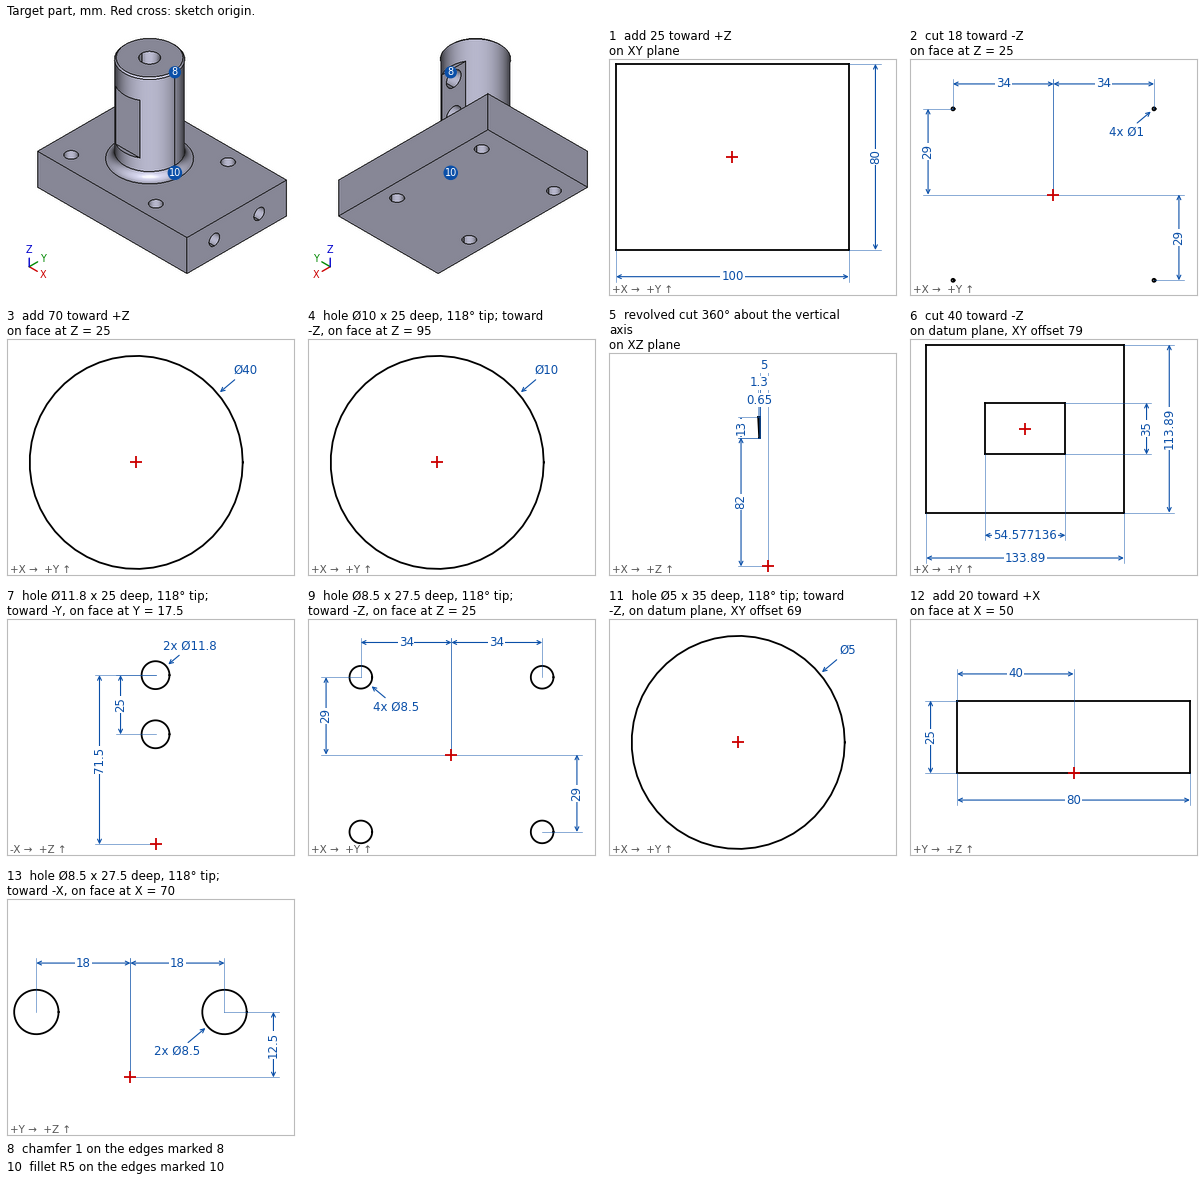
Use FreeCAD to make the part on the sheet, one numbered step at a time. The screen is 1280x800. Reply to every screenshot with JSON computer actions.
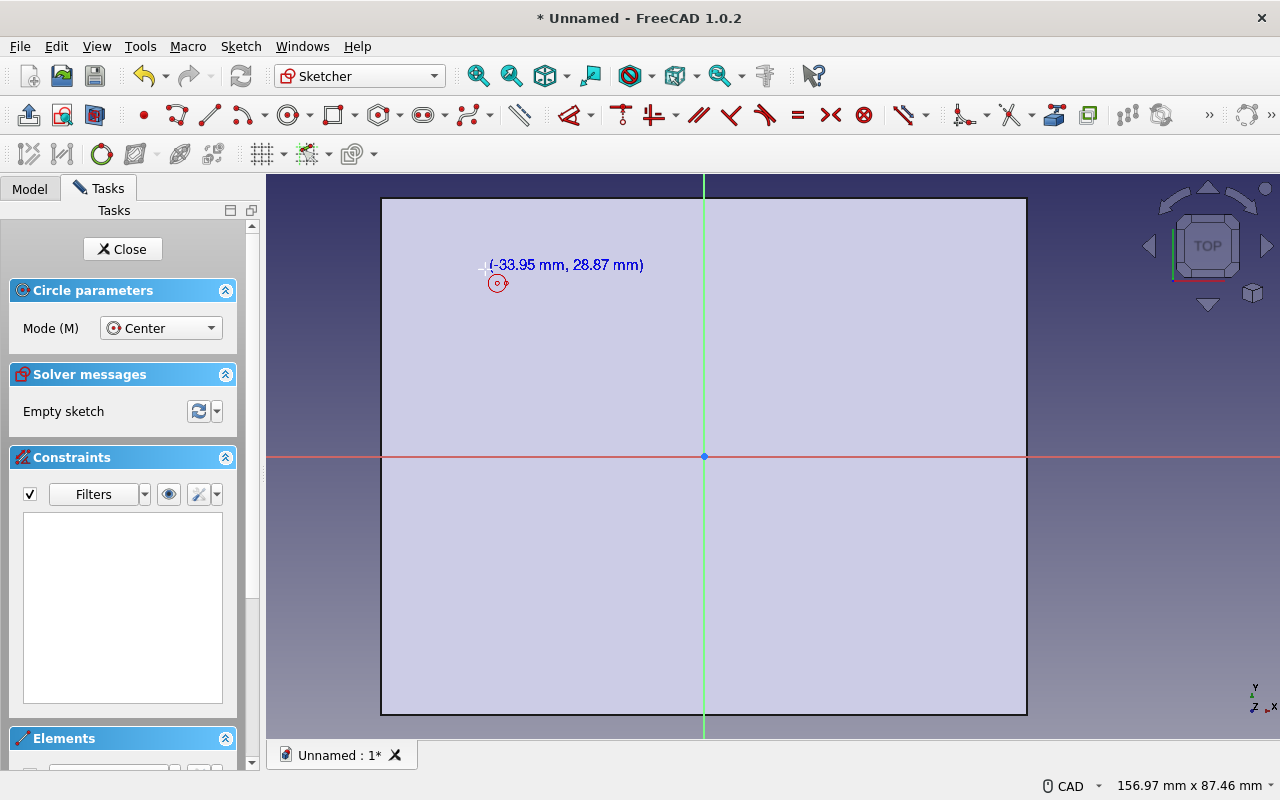
{"action": "left_click", "coordinate": [485, 269]}
{"action": "mouse_move", "coordinate": [487, 267]}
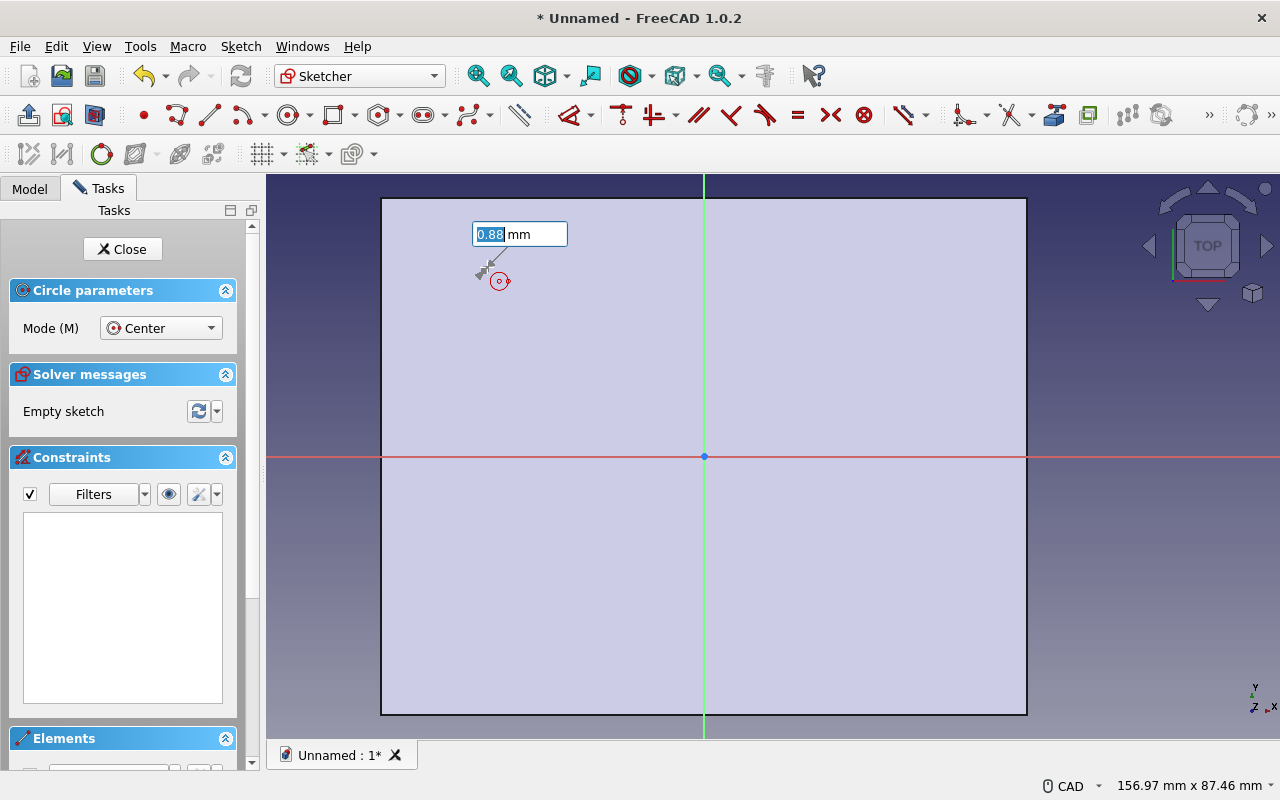
{"action": "type", "text": "1"}
{"action": "key", "text": "Return"}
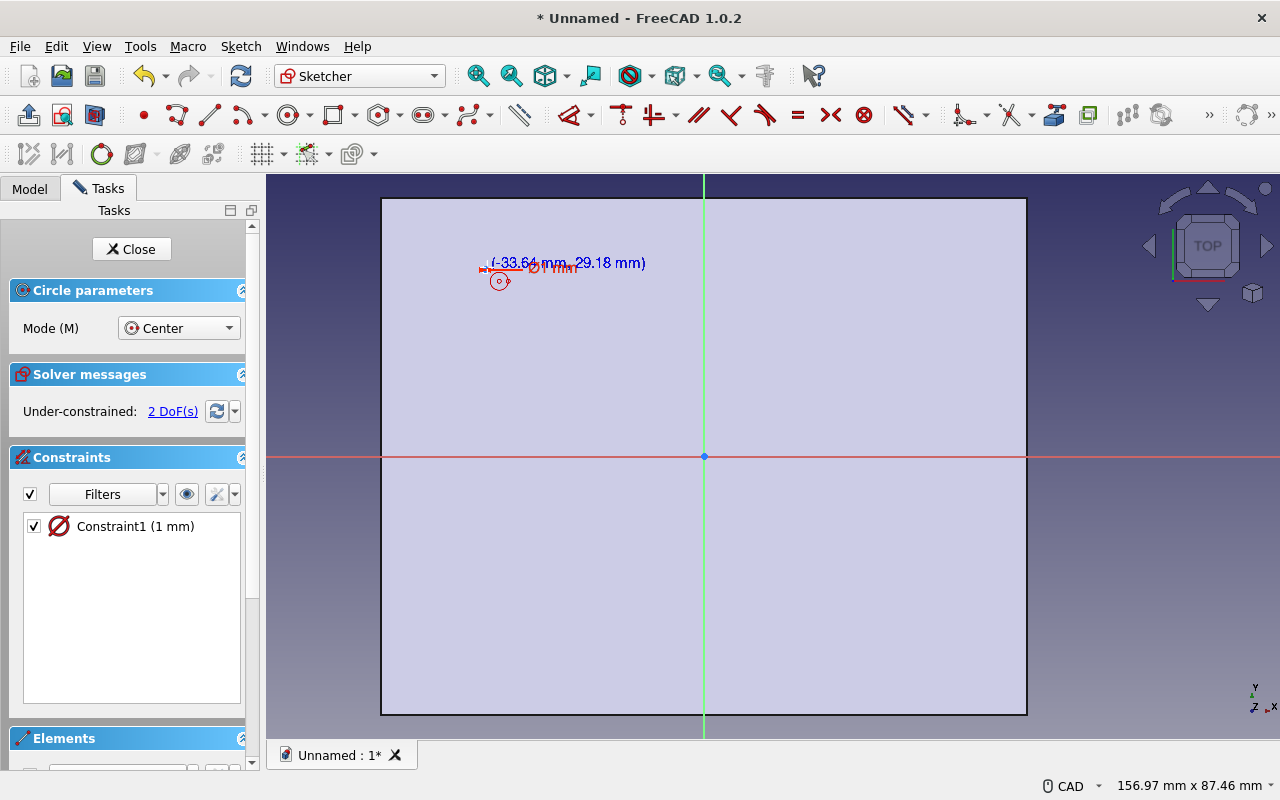
{"action": "scroll", "coordinate": [924, 269], "scroll_direction": "up", "scroll_amount": 10}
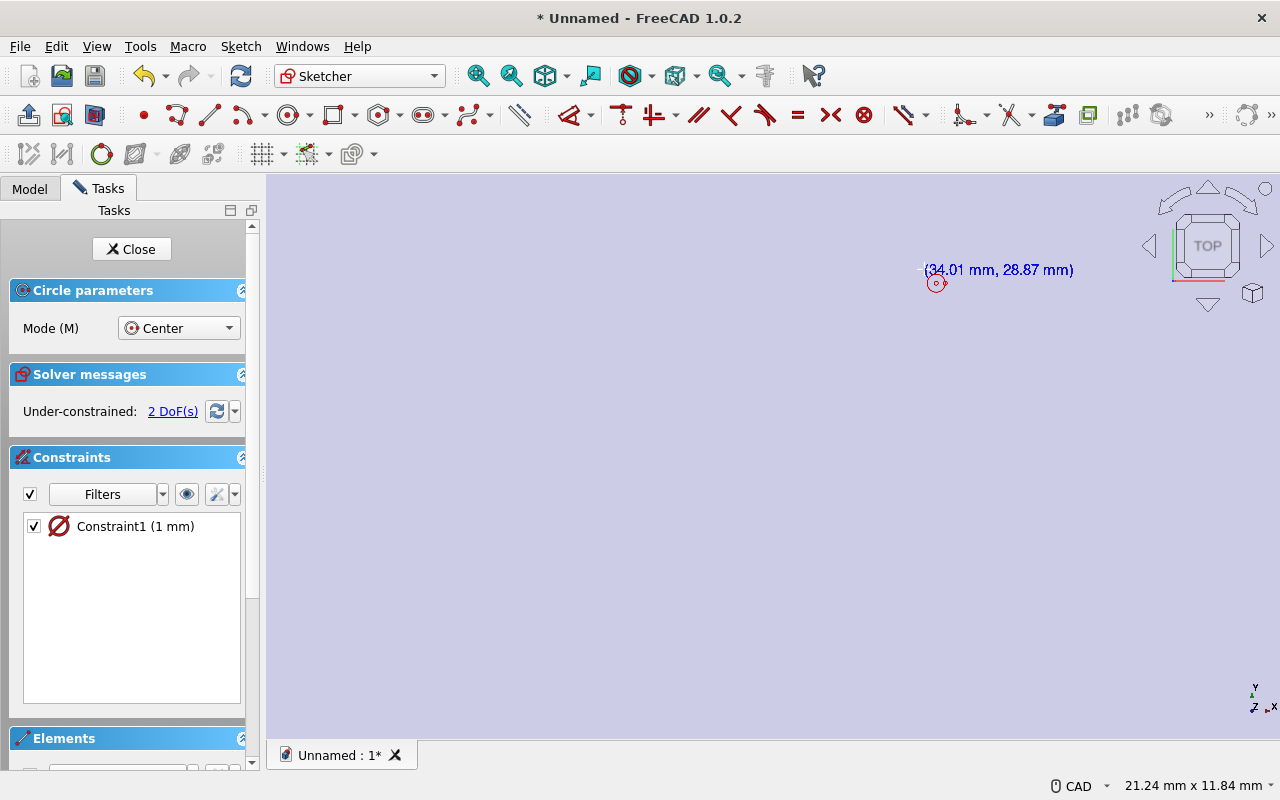
{"action": "scroll", "coordinate": [925, 269], "scroll_direction": "down", "scroll_amount": 10}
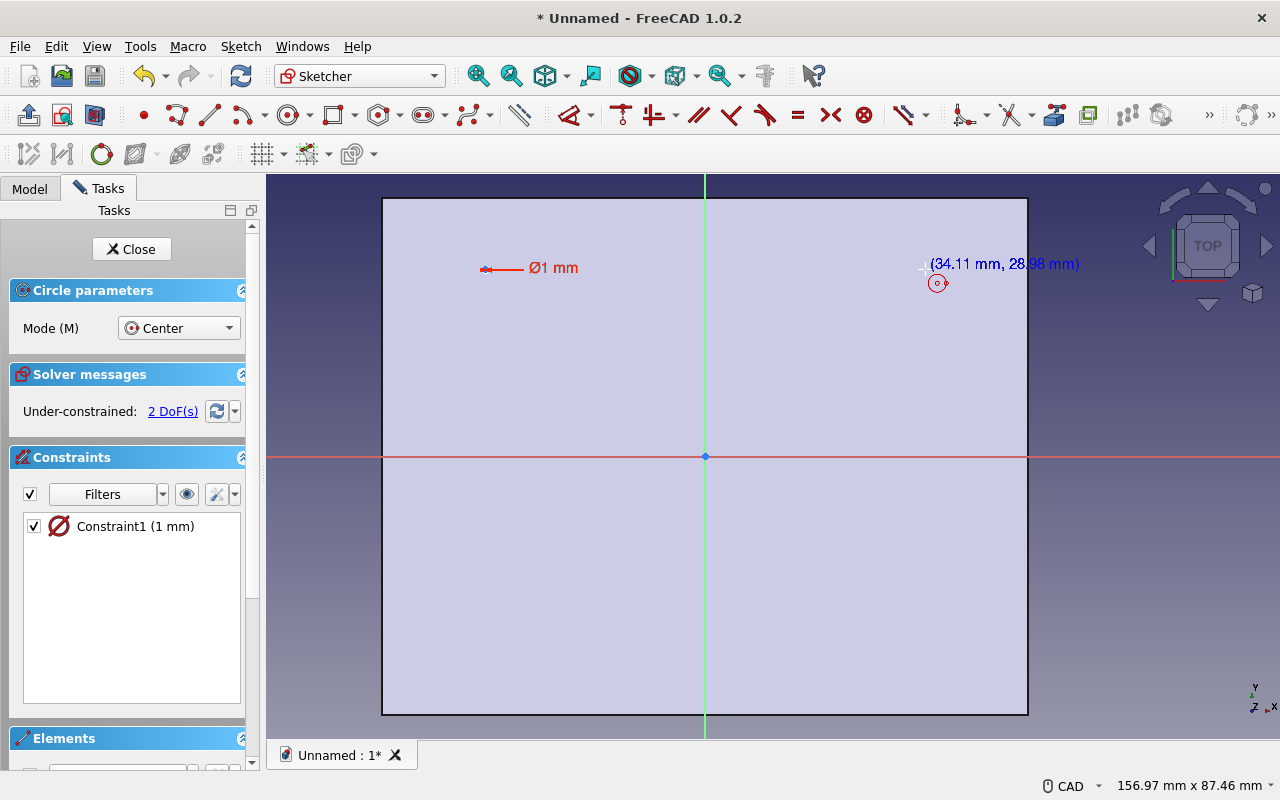
{"action": "left_click", "coordinate": [925, 269]}
{"action": "mouse_move", "coordinate": [927, 267]}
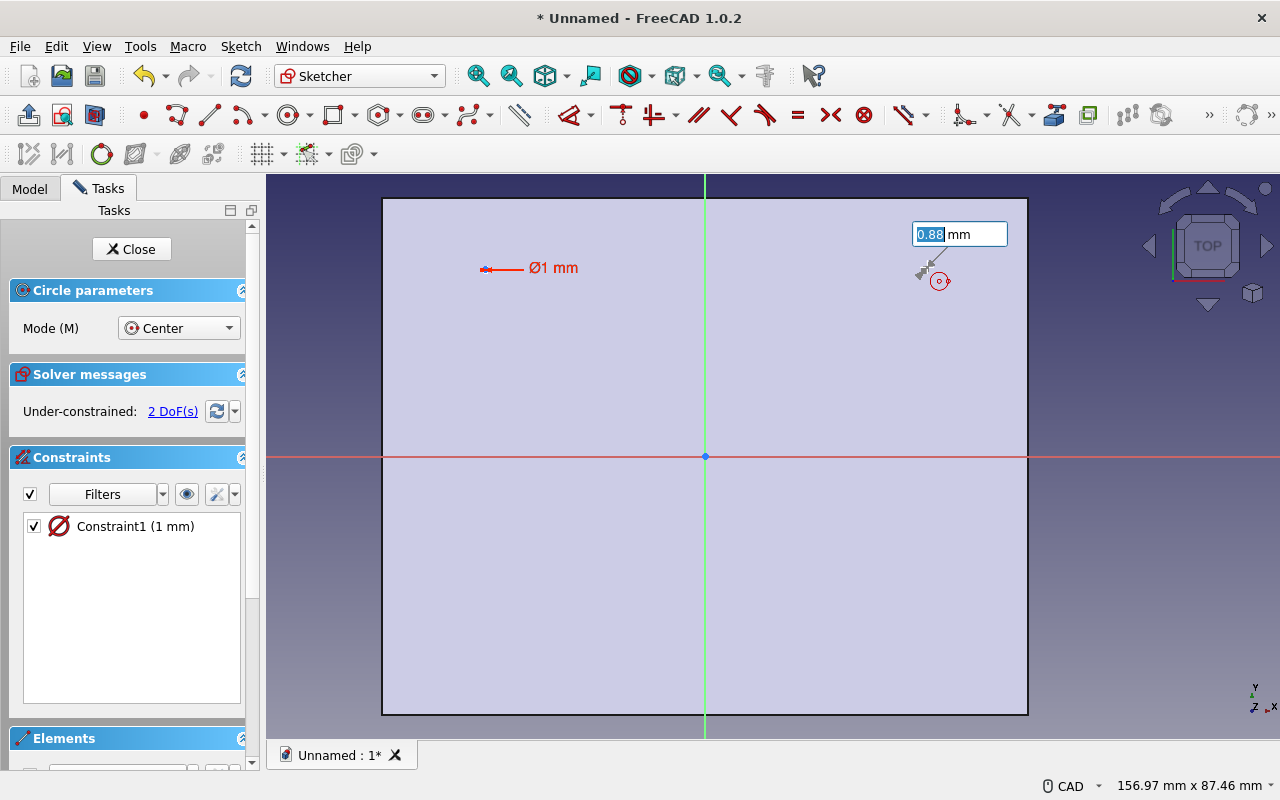
{"action": "type", "text": "1"}
{"action": "key", "text": "Return"}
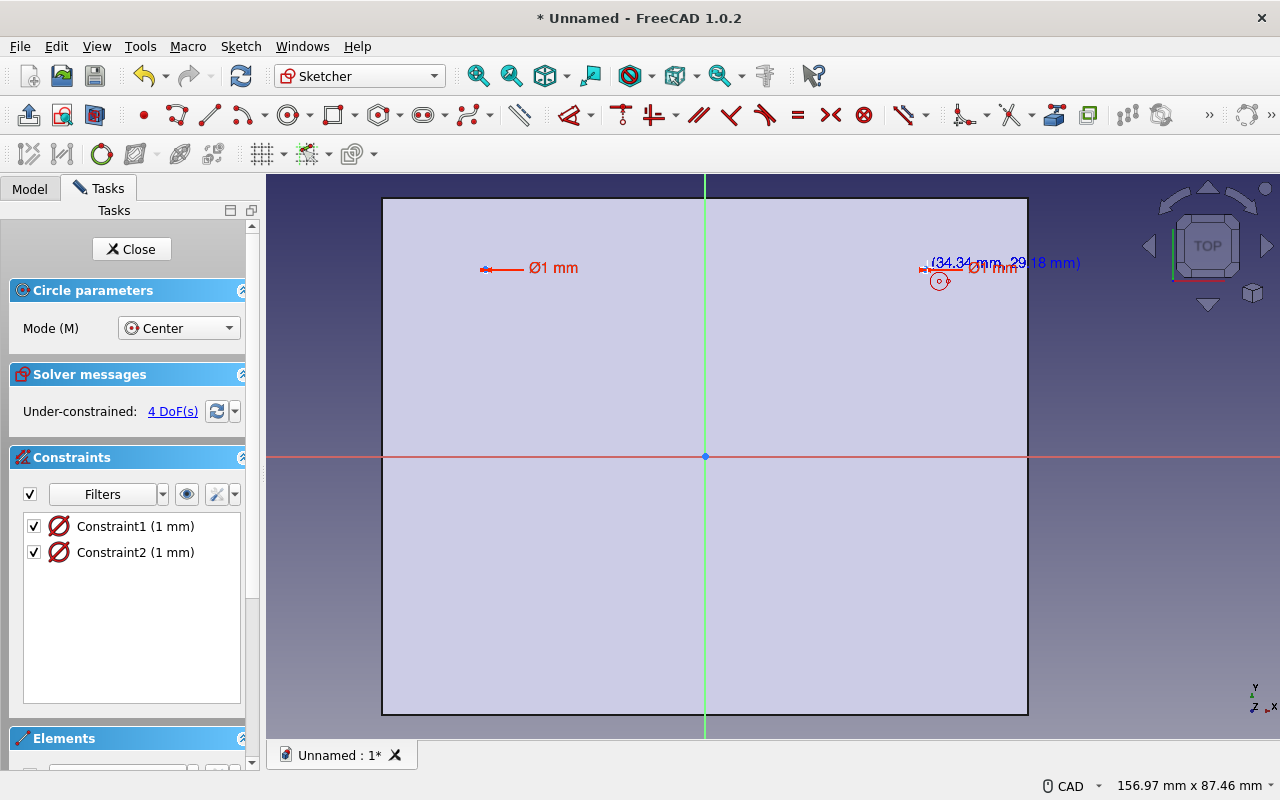
{"action": "scroll", "coordinate": [925, 644], "scroll_direction": "up", "scroll_amount": 10}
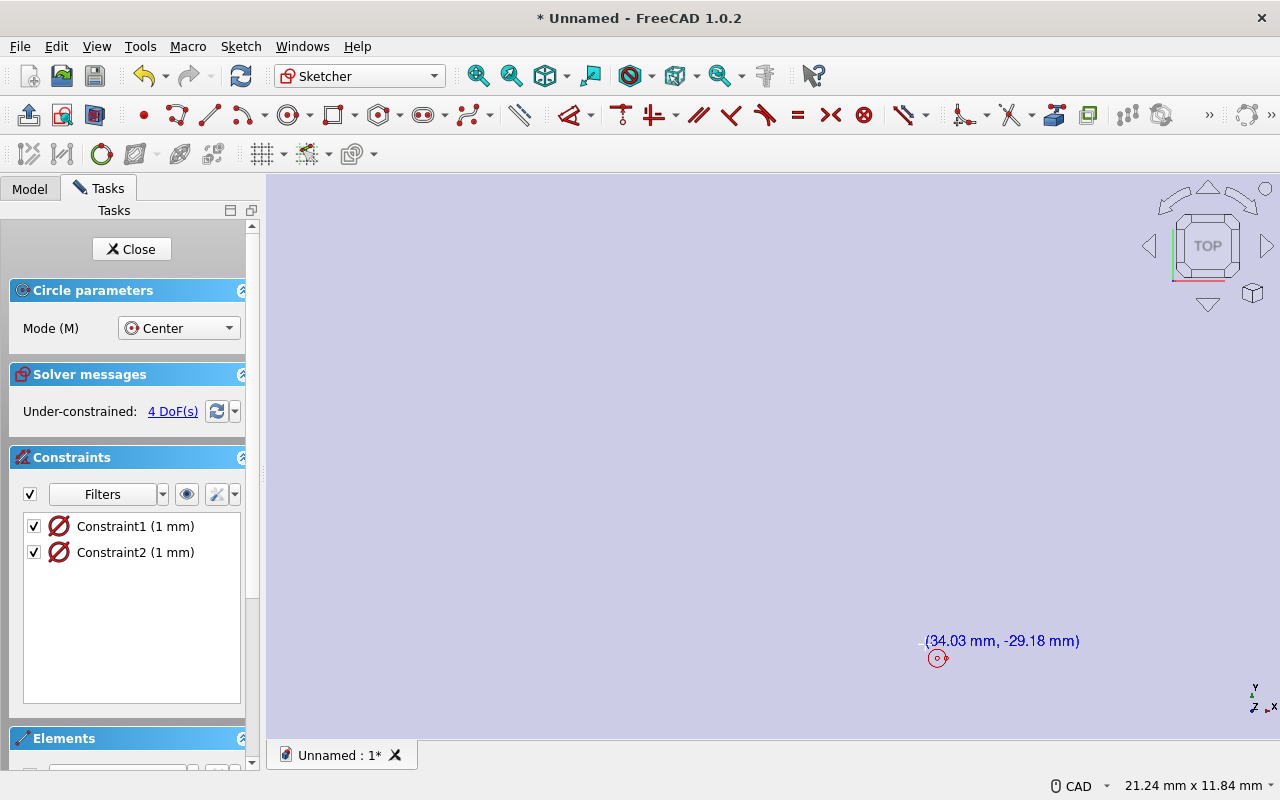
{"action": "scroll", "coordinate": [925, 645], "scroll_direction": "down", "scroll_amount": 10}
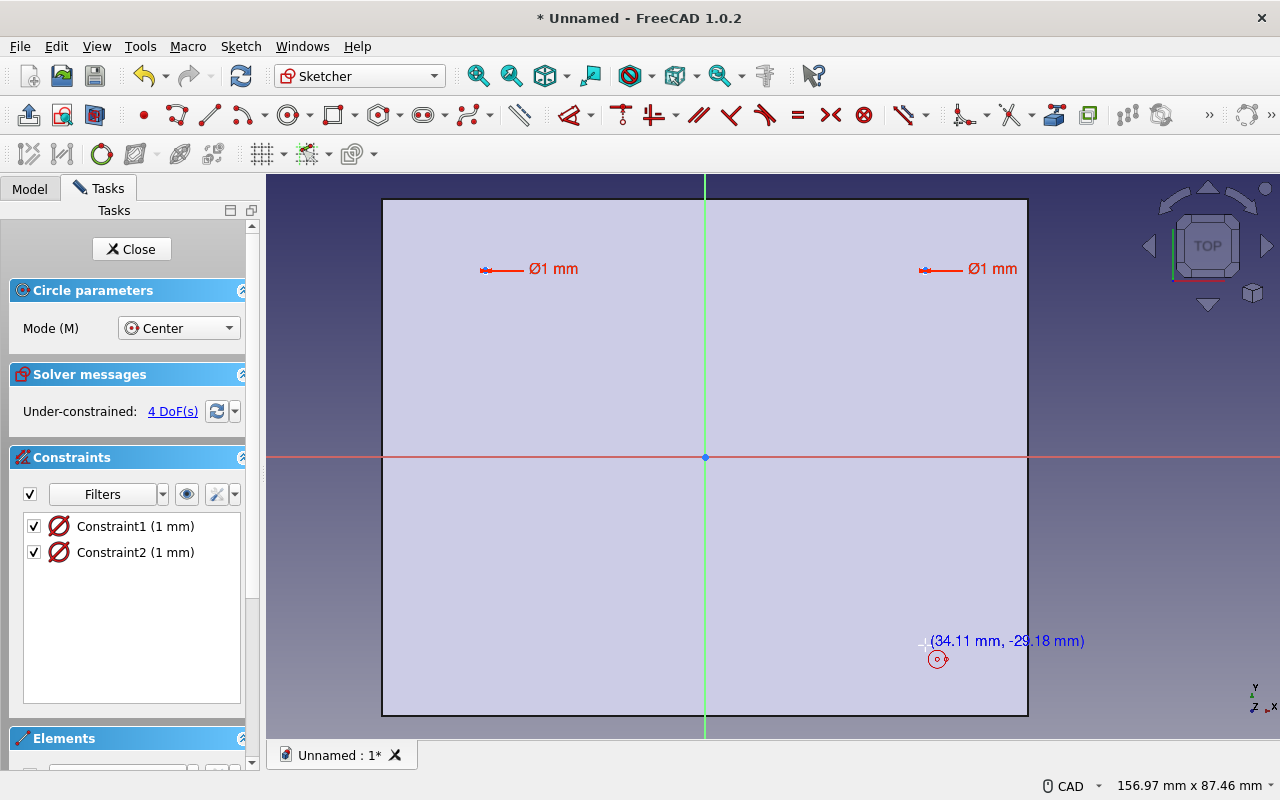
{"action": "left_click", "coordinate": [925, 645]}
{"action": "mouse_move", "coordinate": [927, 642]}